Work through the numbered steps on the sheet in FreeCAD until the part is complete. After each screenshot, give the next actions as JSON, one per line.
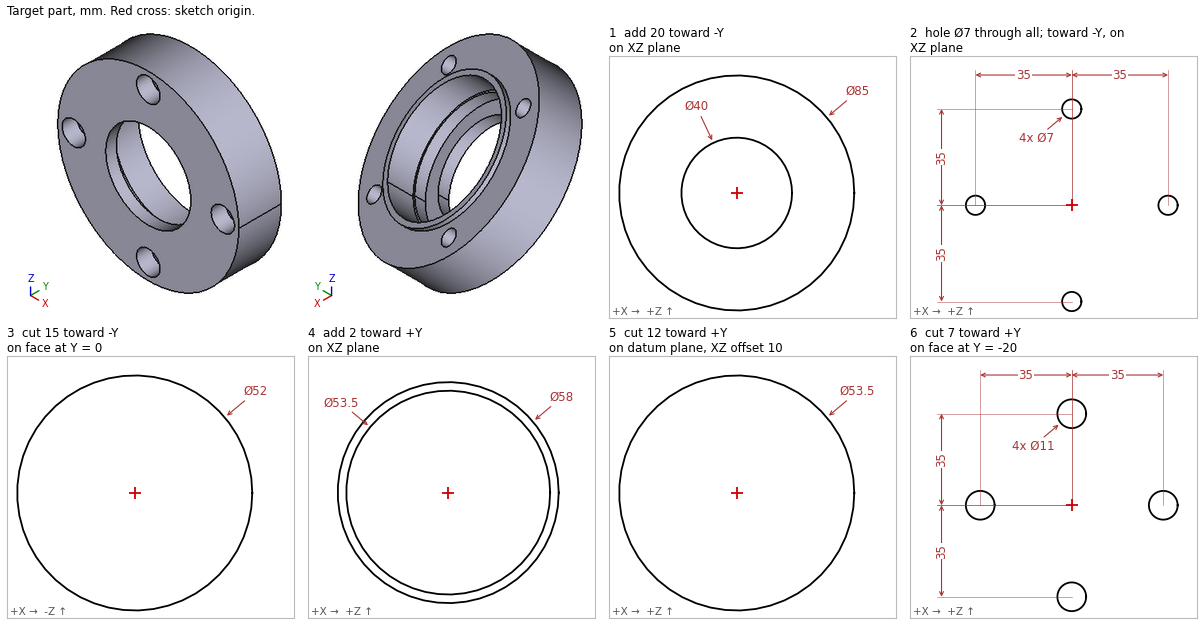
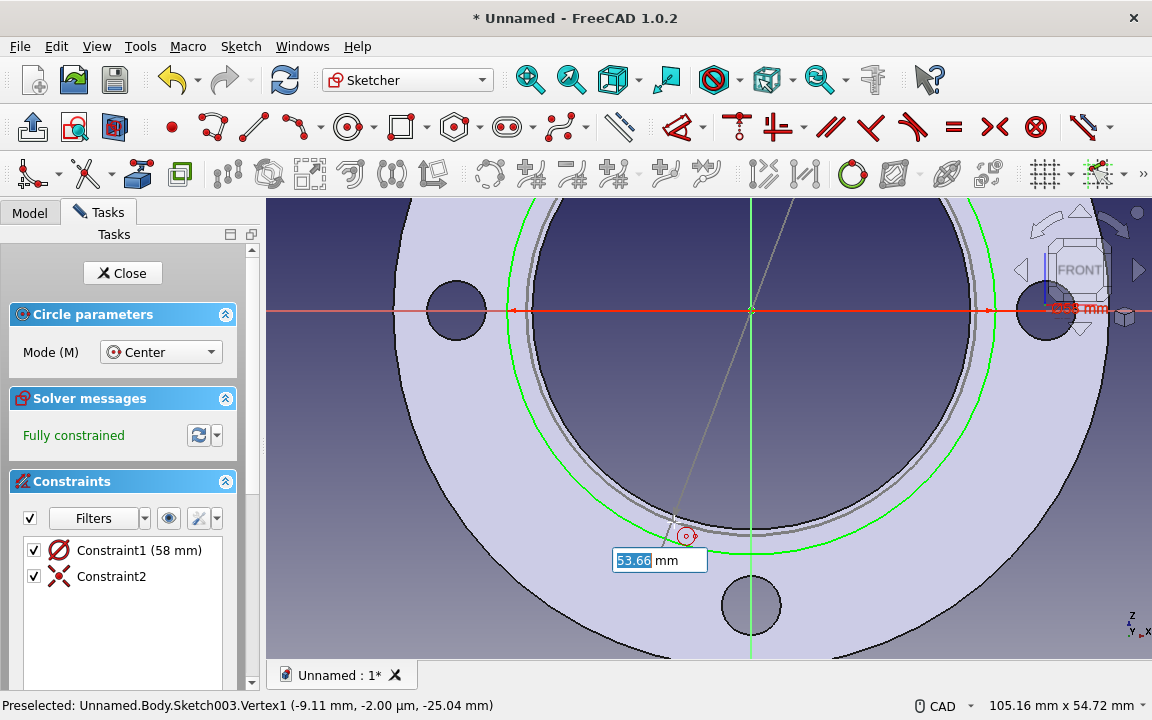
{"action": "type", "text": "53.5"}
{"action": "key", "text": "Return"}
{"action": "key", "text": "Escape"}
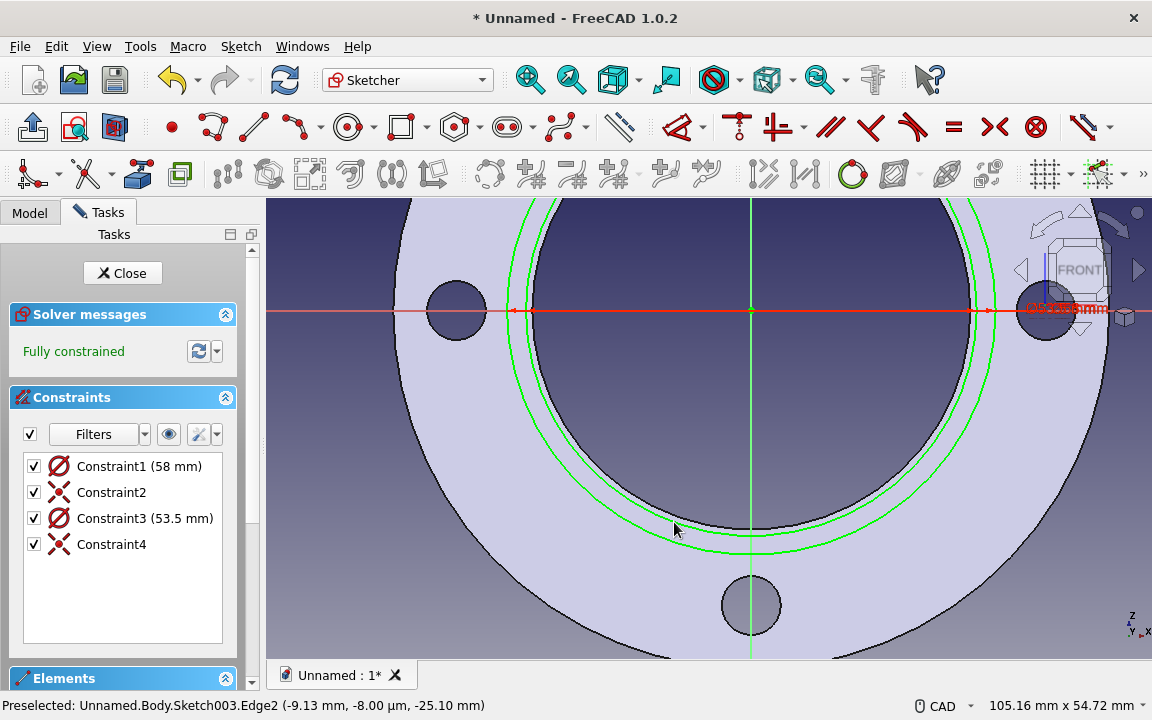
{"action": "left_click", "coordinate": [123, 273]}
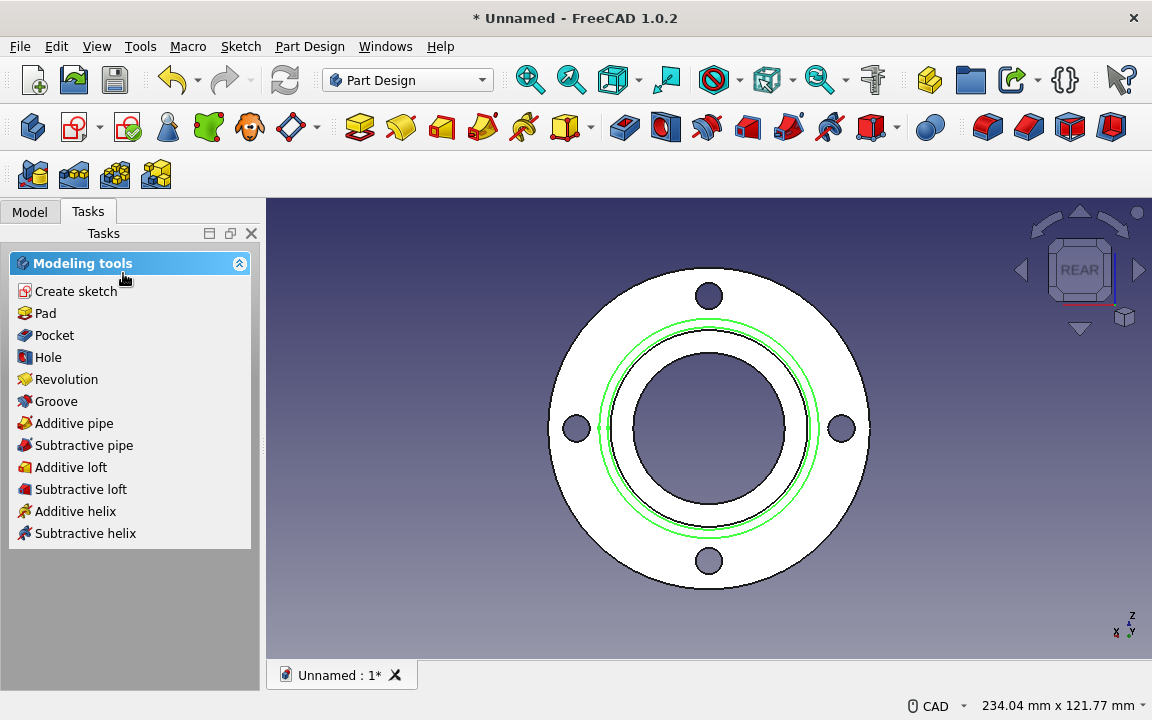
{"action": "left_click", "coordinate": [360, 128]}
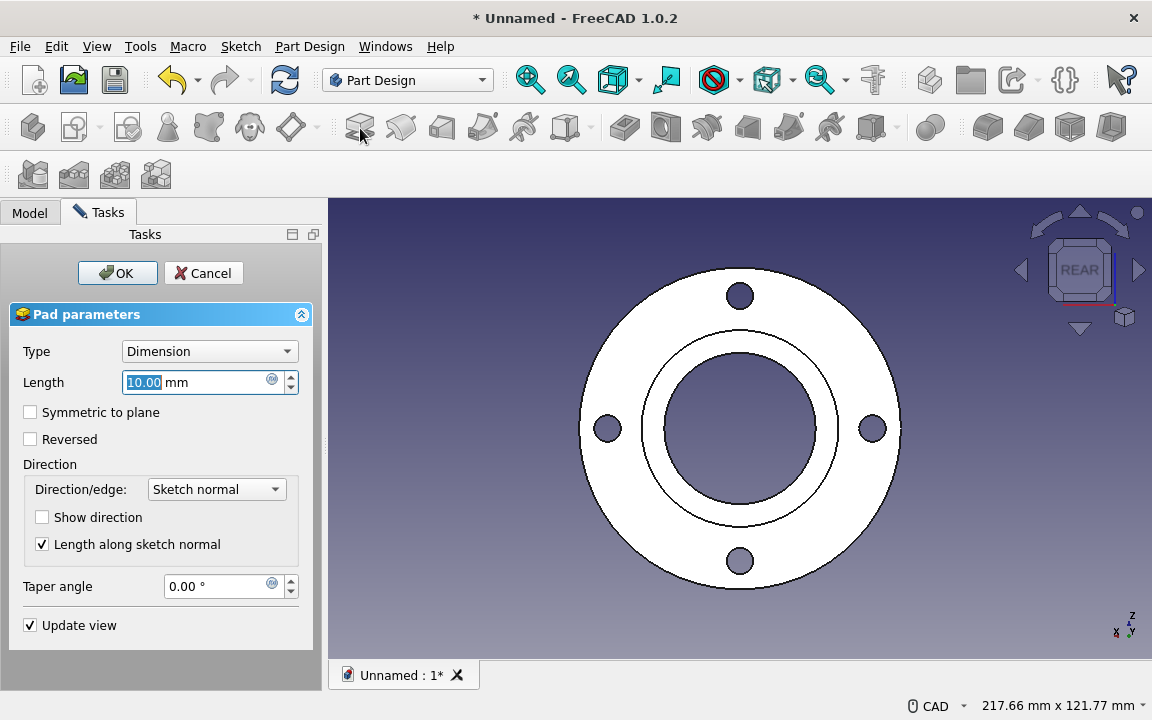
{"action": "type", "text": "2"}
{"action": "key", "text": "Tab"}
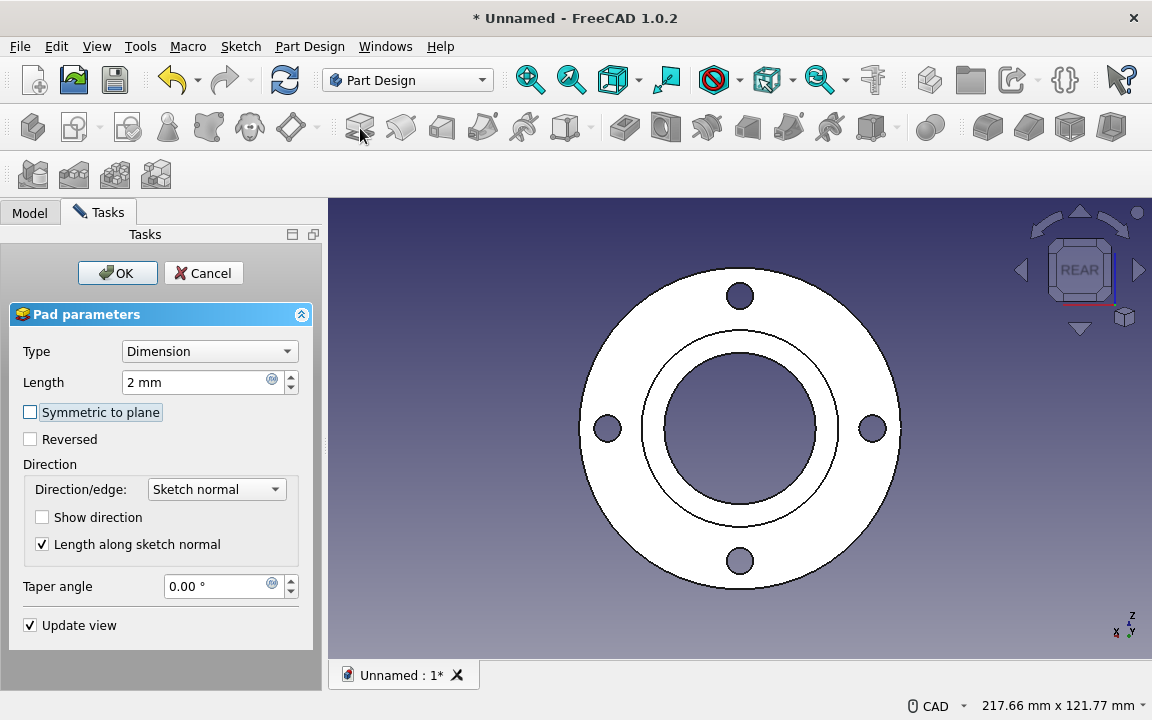
{"action": "left_click", "coordinate": [31, 439]}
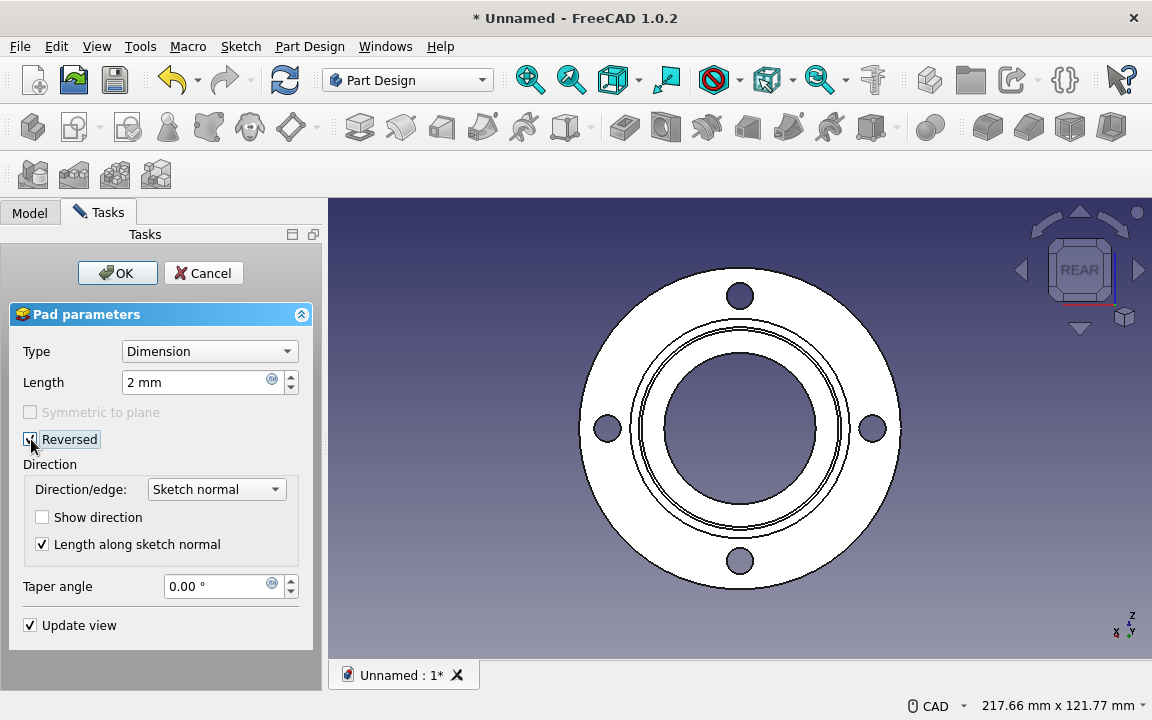
{"action": "left_click", "coordinate": [118, 273]}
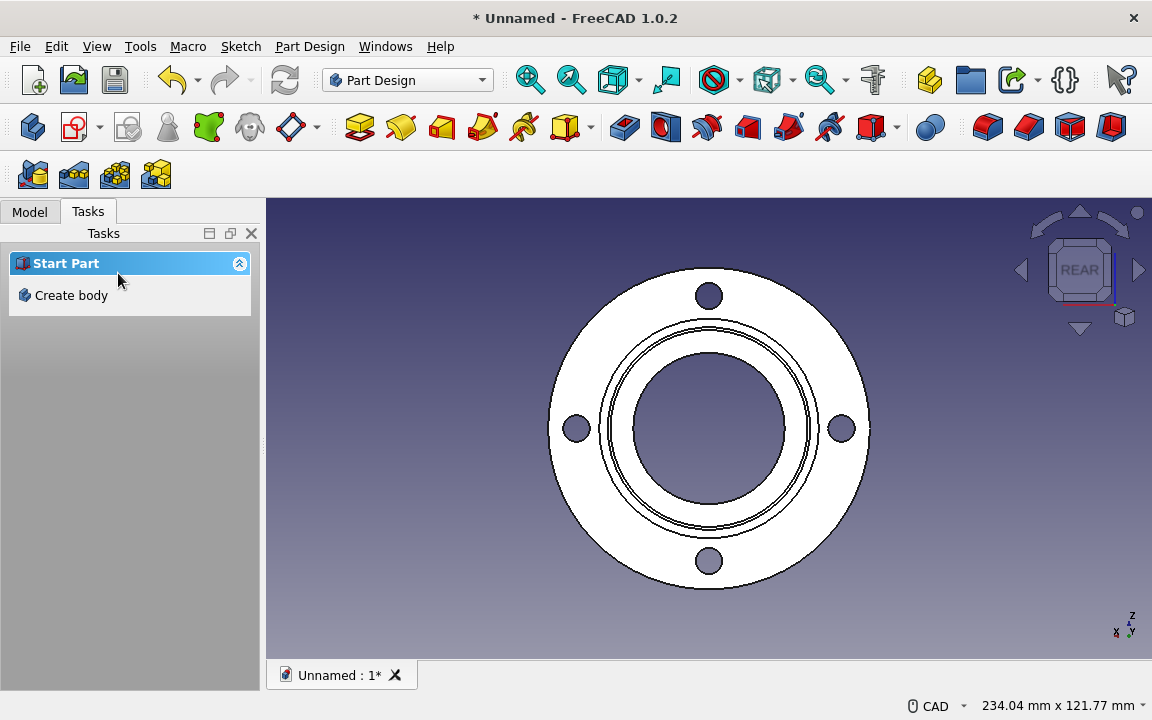
{"action": "left_click", "coordinate": [30, 212]}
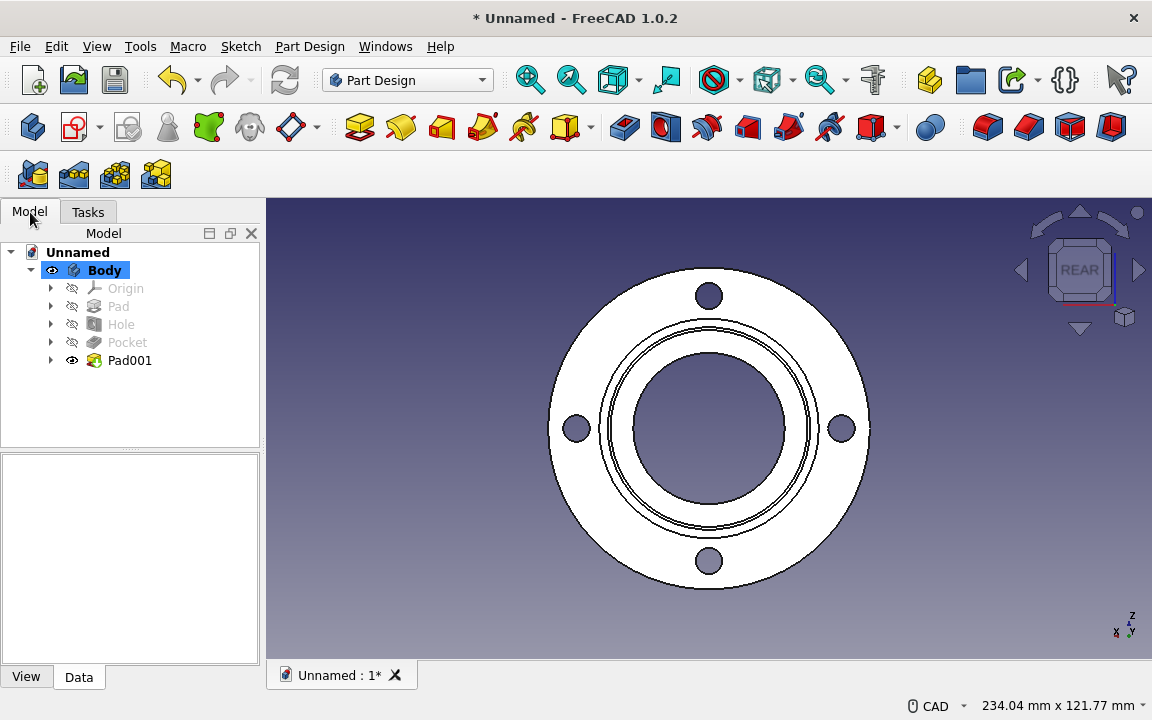
{"action": "left_click", "coordinate": [51, 288]}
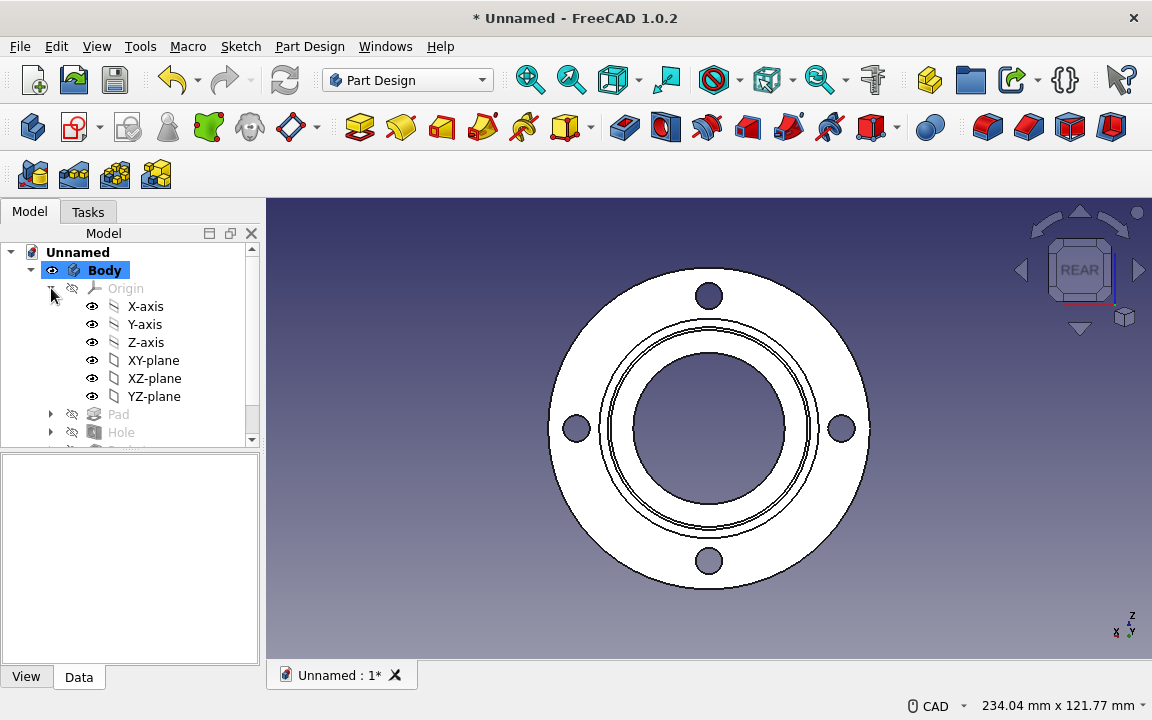
{"action": "left_click", "coordinate": [137, 378]}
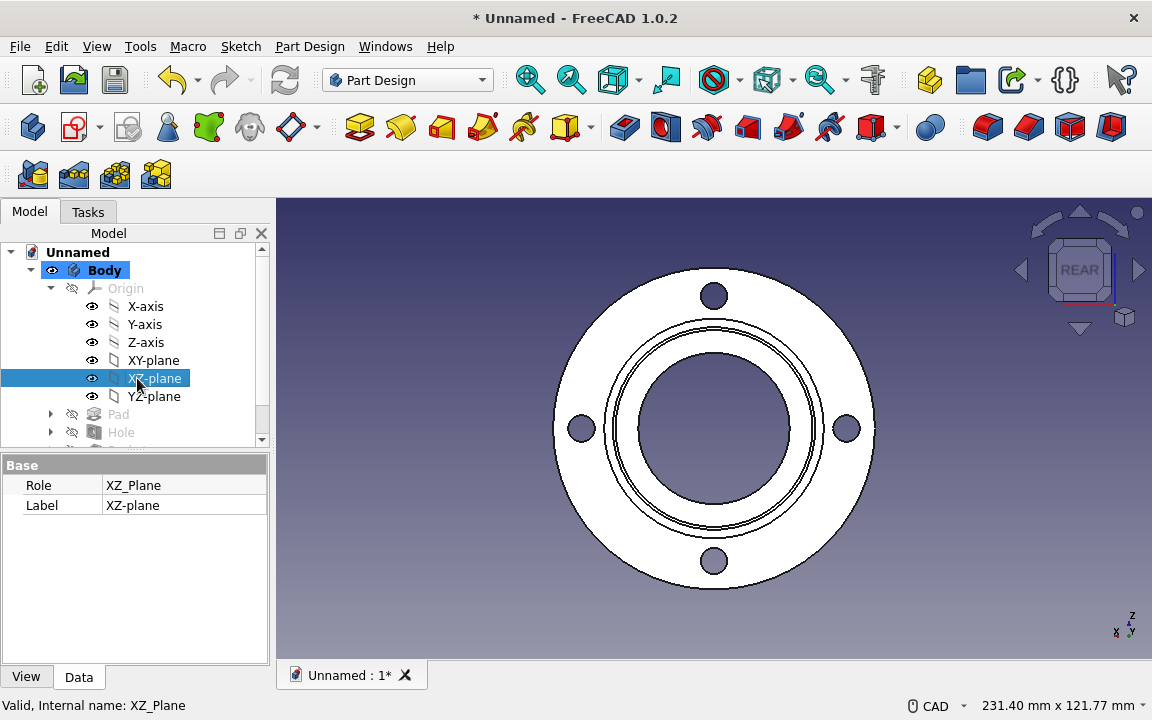
{"action": "left_click", "coordinate": [290, 128]}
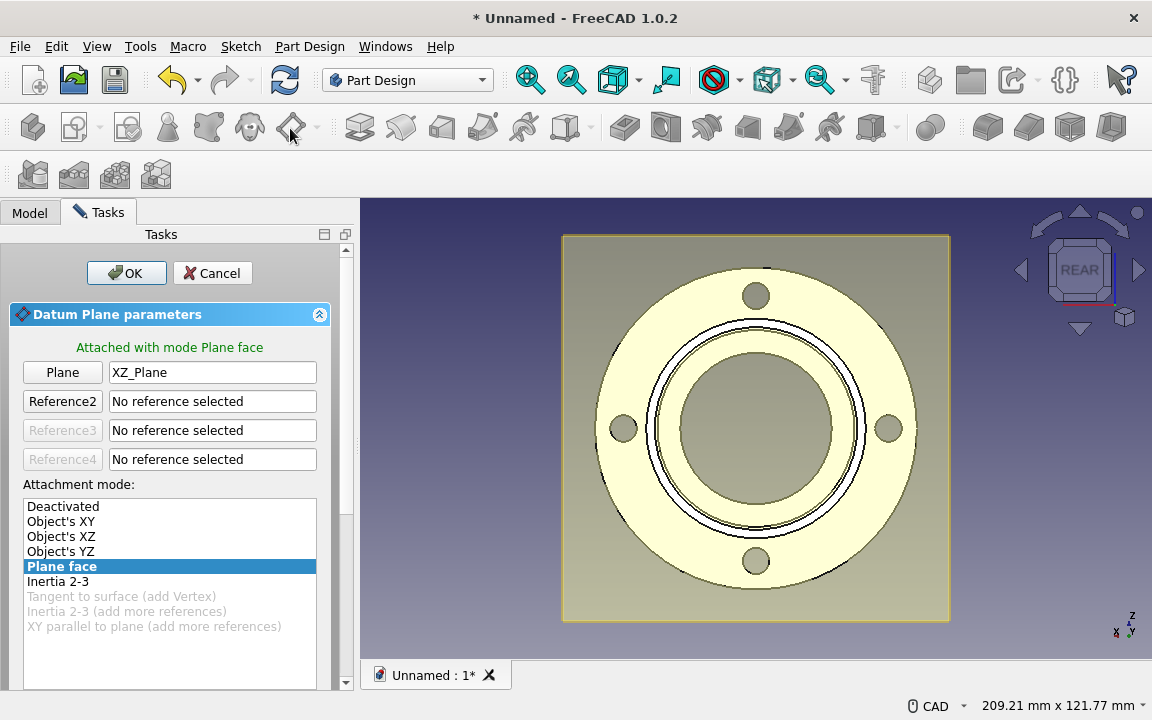
{"action": "scroll", "coordinate": [346, 467], "scroll_direction": "down", "scroll_amount": 4}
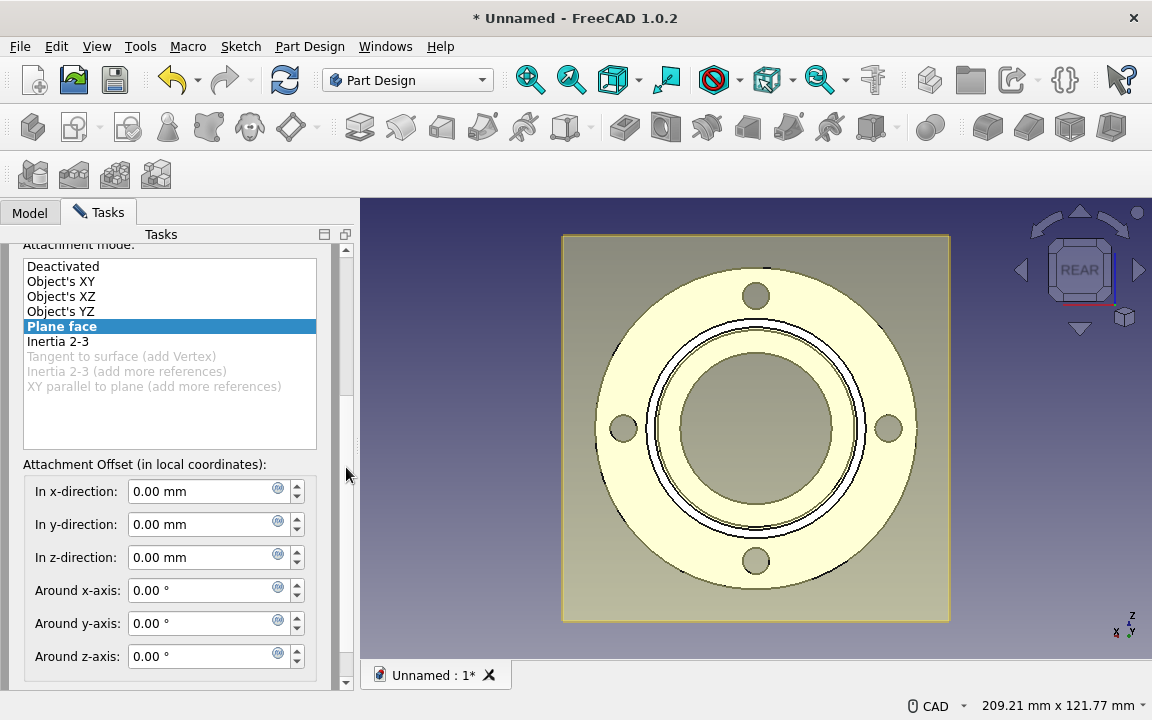
{"action": "triple_click", "coordinate": [210, 558]}